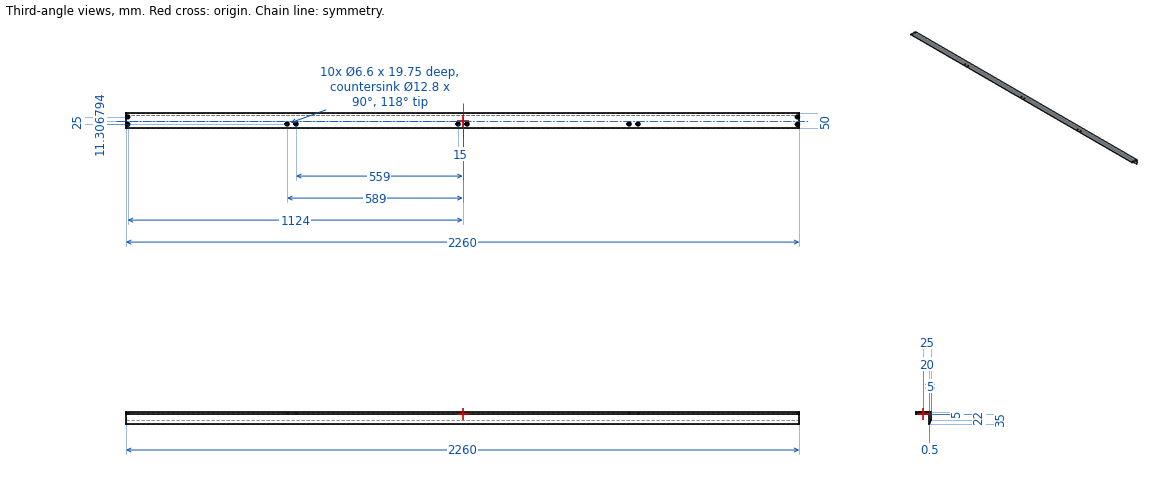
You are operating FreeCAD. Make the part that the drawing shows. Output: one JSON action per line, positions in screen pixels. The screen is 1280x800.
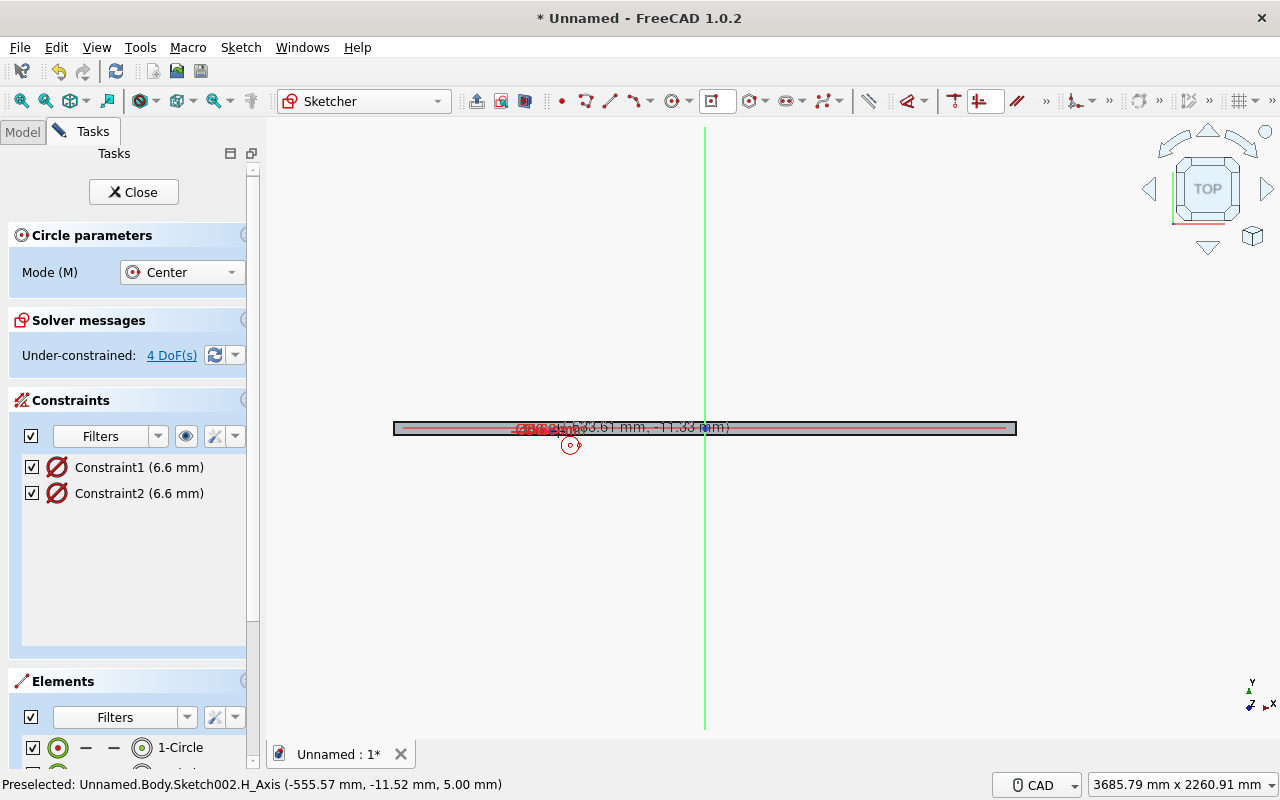
{"action": "scroll", "coordinate": [701, 432], "scroll_direction": "up", "scroll_amount": 17}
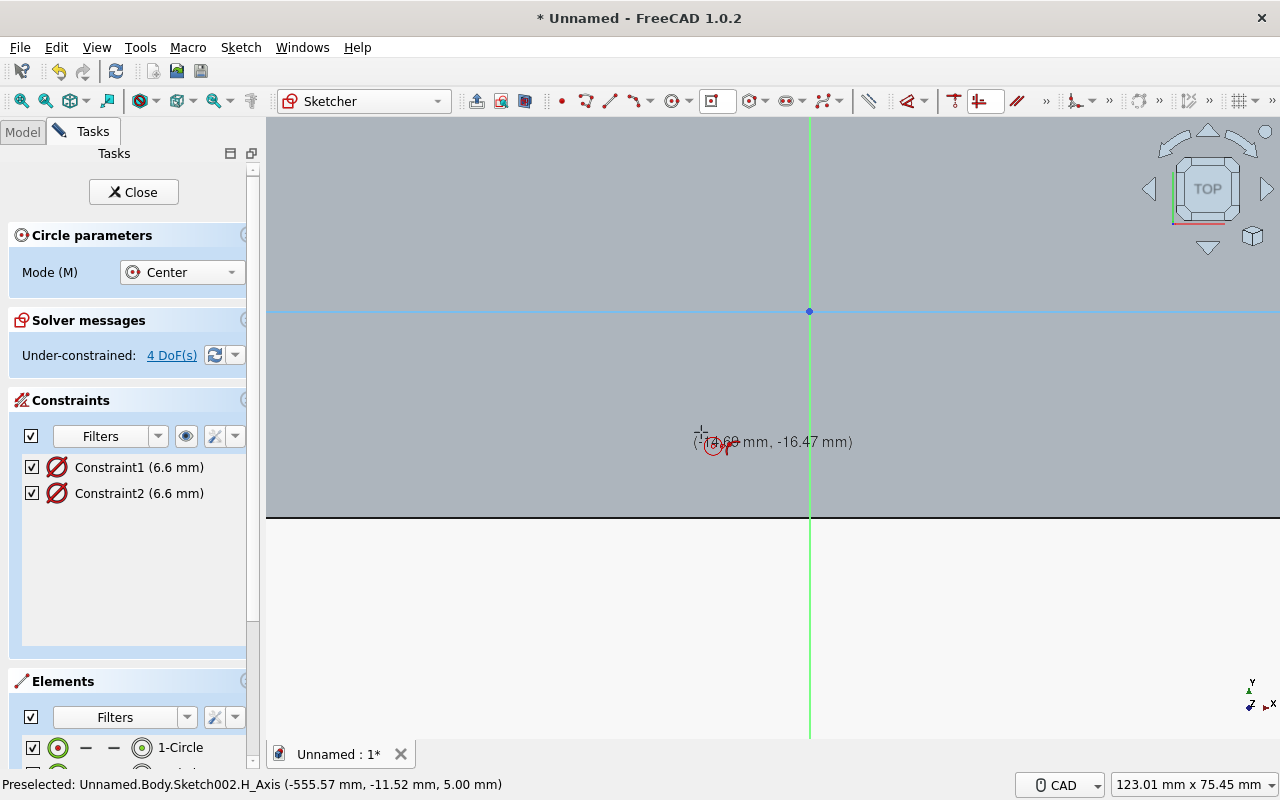
{"action": "scroll", "coordinate": [700, 433], "scroll_direction": "down", "scroll_amount": 16}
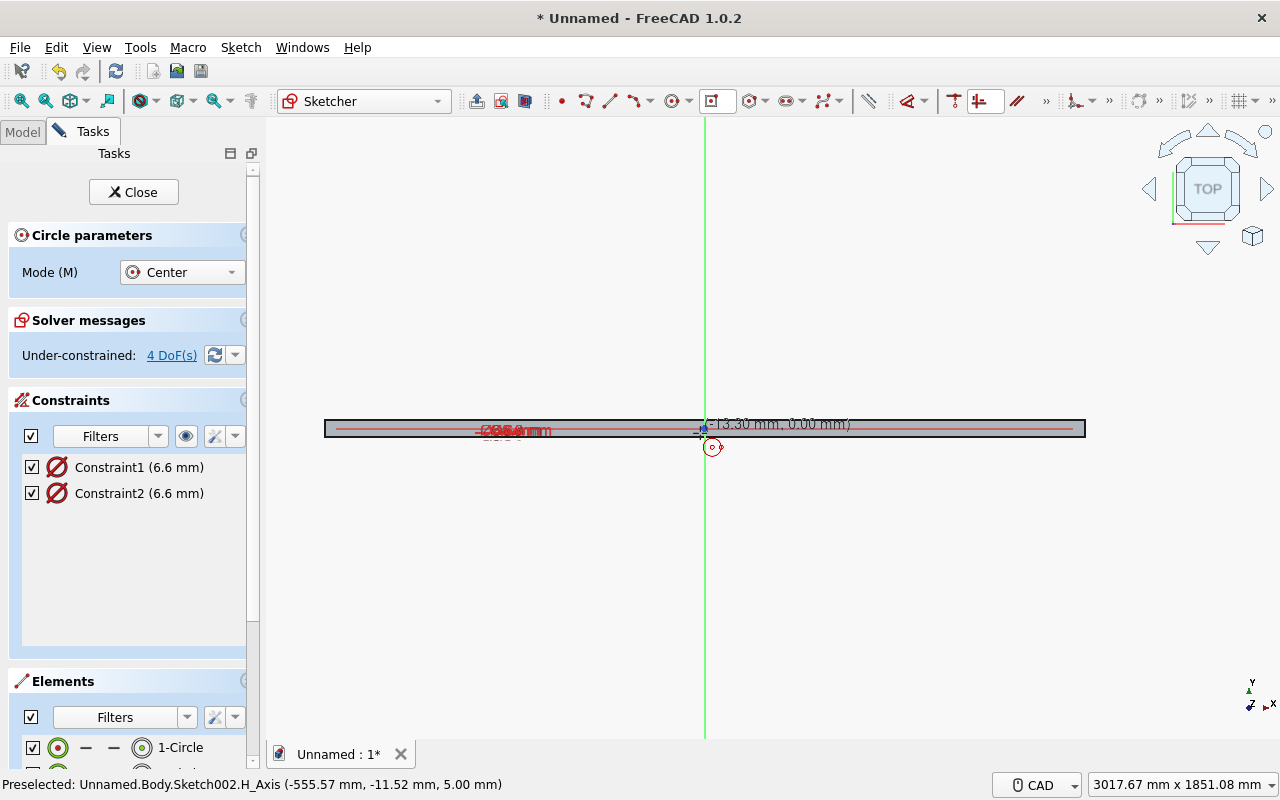
{"action": "scroll", "coordinate": [700, 432], "scroll_direction": "up", "scroll_amount": 8}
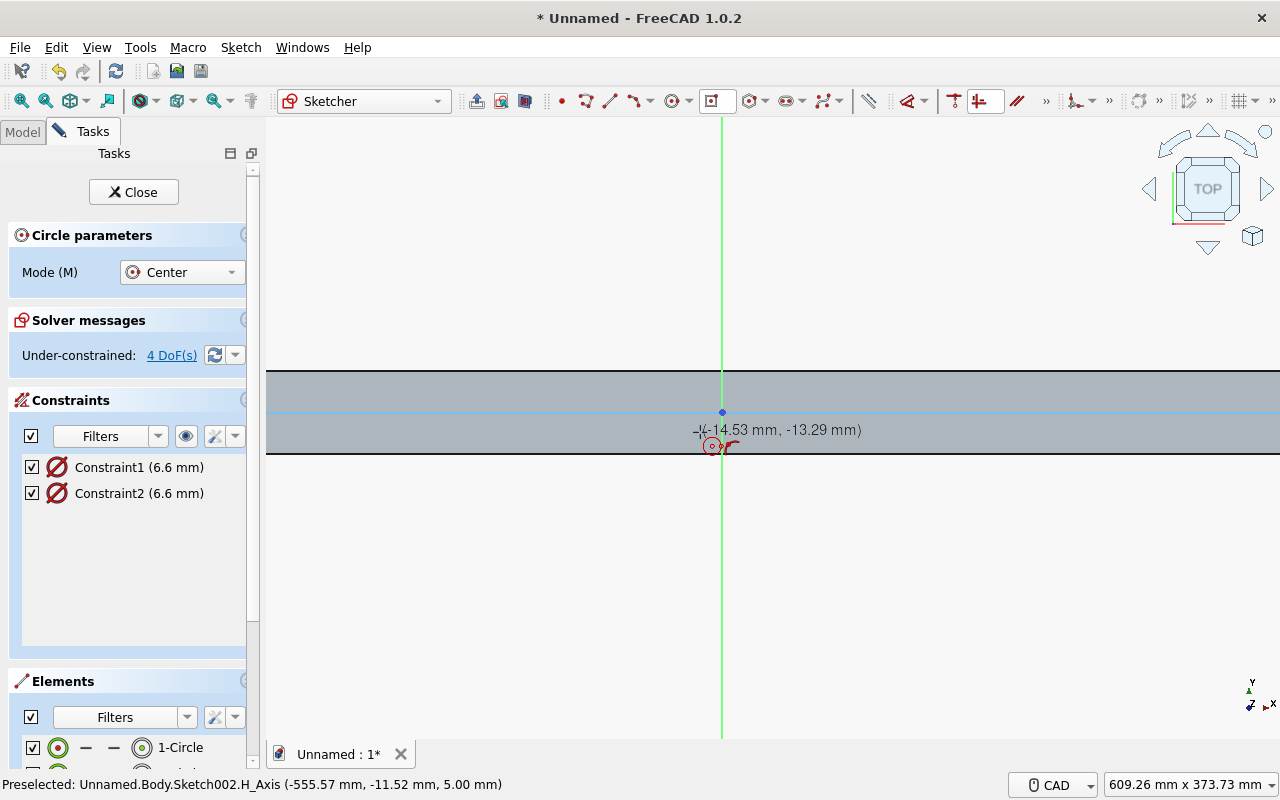
{"action": "left_click", "coordinate": [698, 432]}
{"action": "mouse_move", "coordinate": [701, 428]}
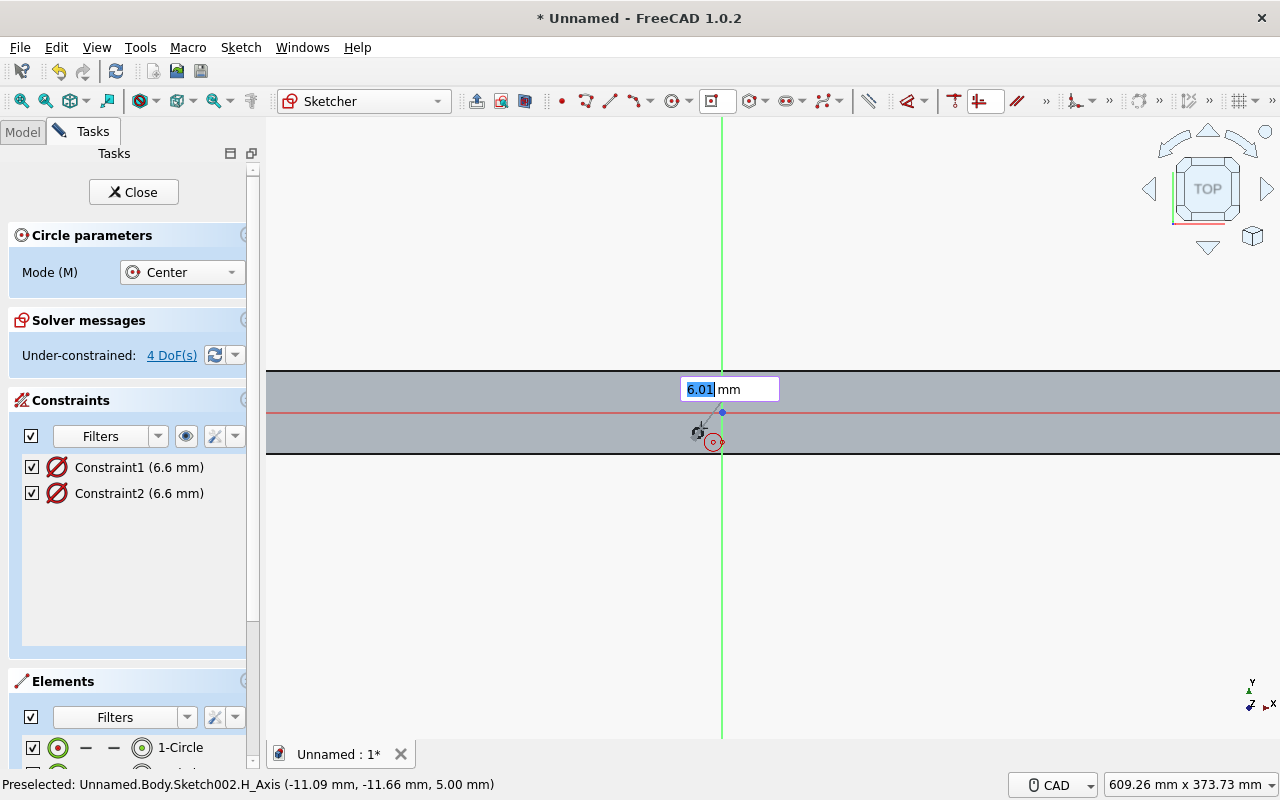
{"action": "type", "text": "6.6"}
{"action": "key", "text": "Return"}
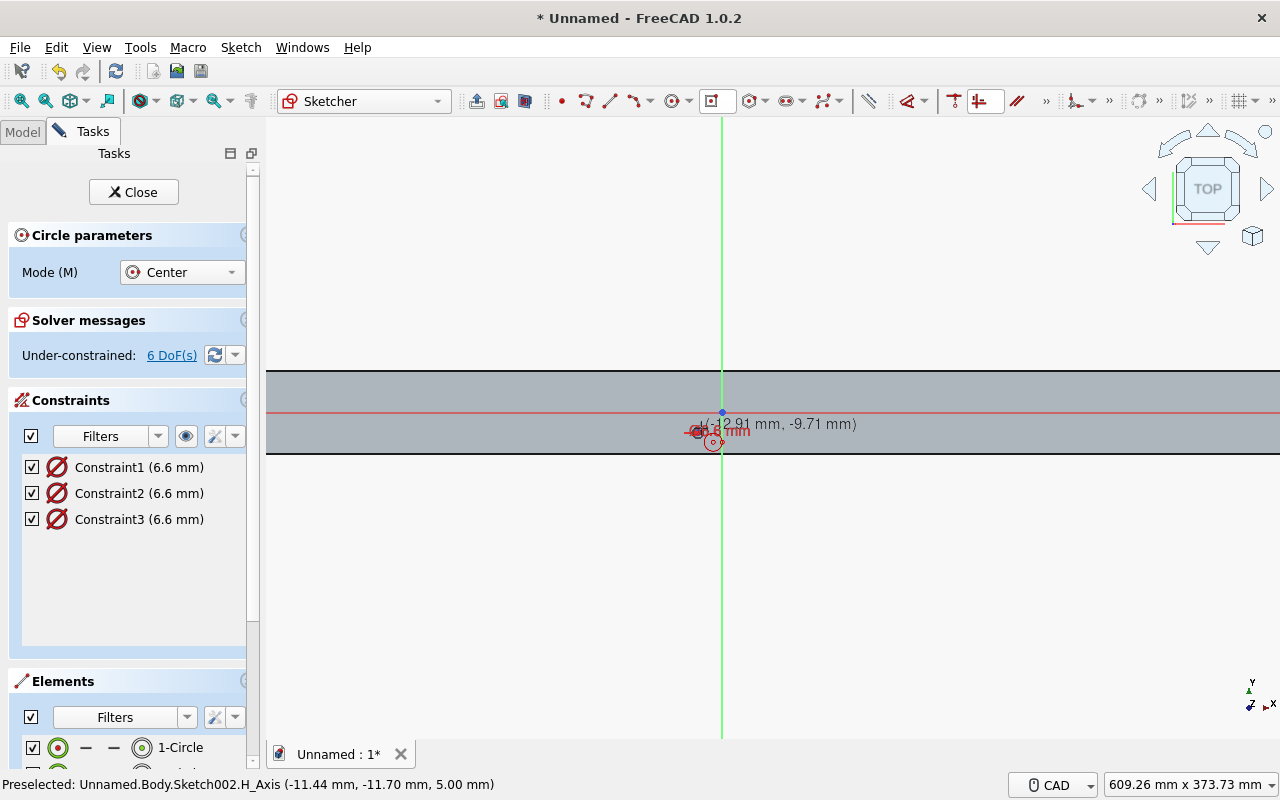
{"action": "scroll", "coordinate": [747, 432], "scroll_direction": "up", "scroll_amount": 8}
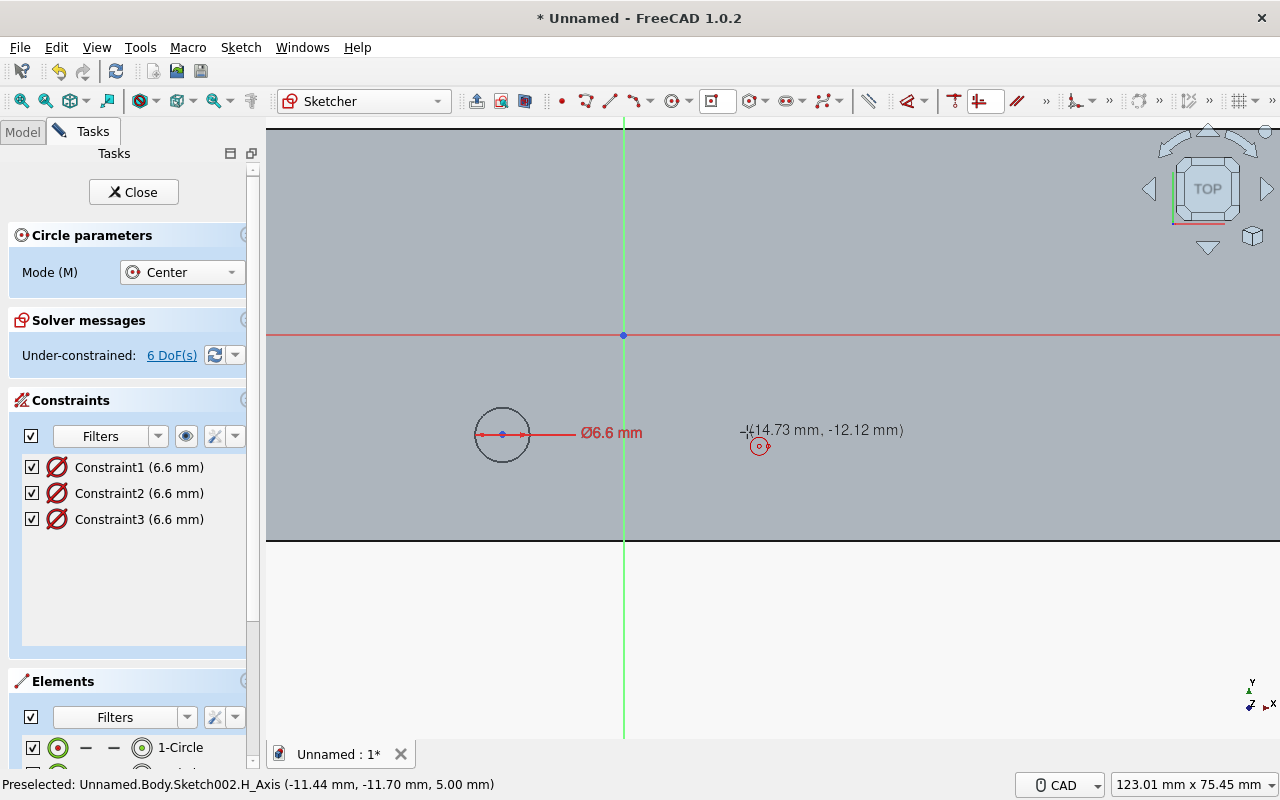
{"action": "scroll", "coordinate": [708, 432], "scroll_direction": "down", "scroll_amount": 16}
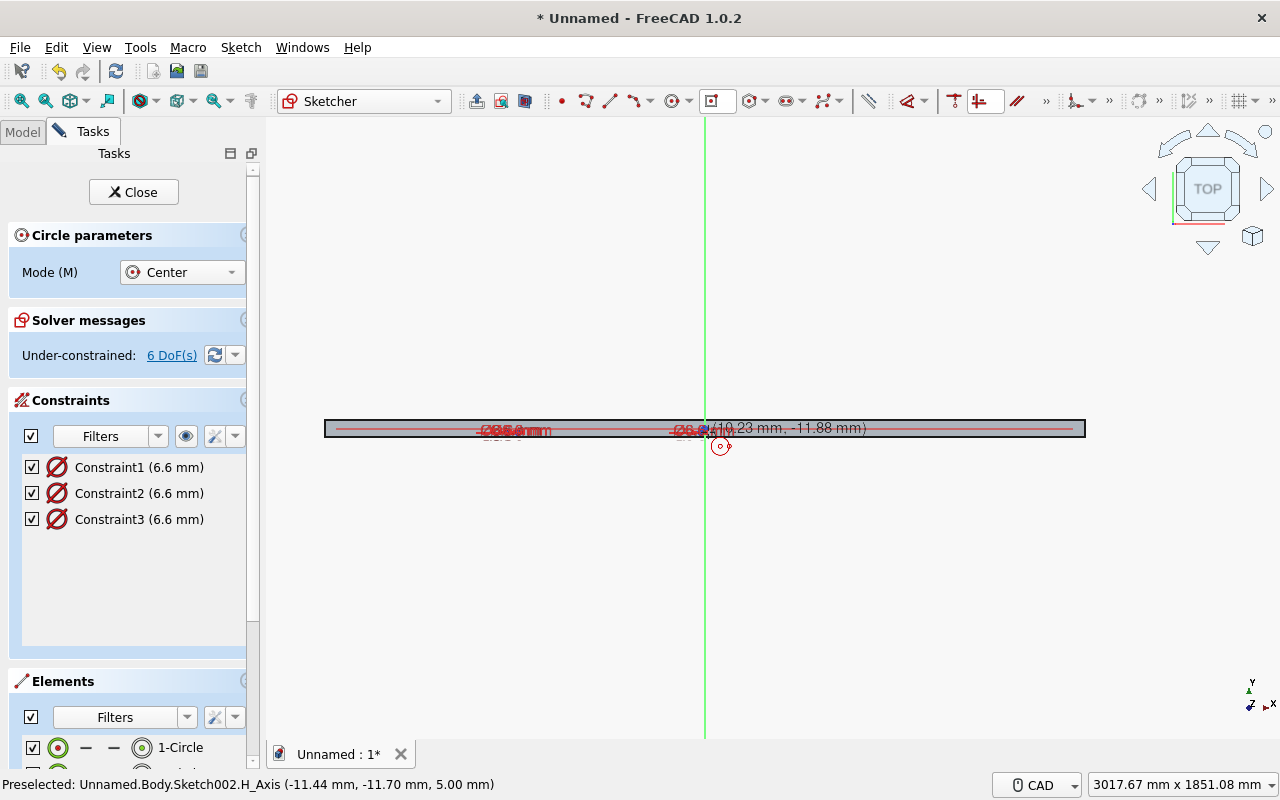
{"action": "scroll", "coordinate": [710, 432], "scroll_direction": "up", "scroll_amount": 8}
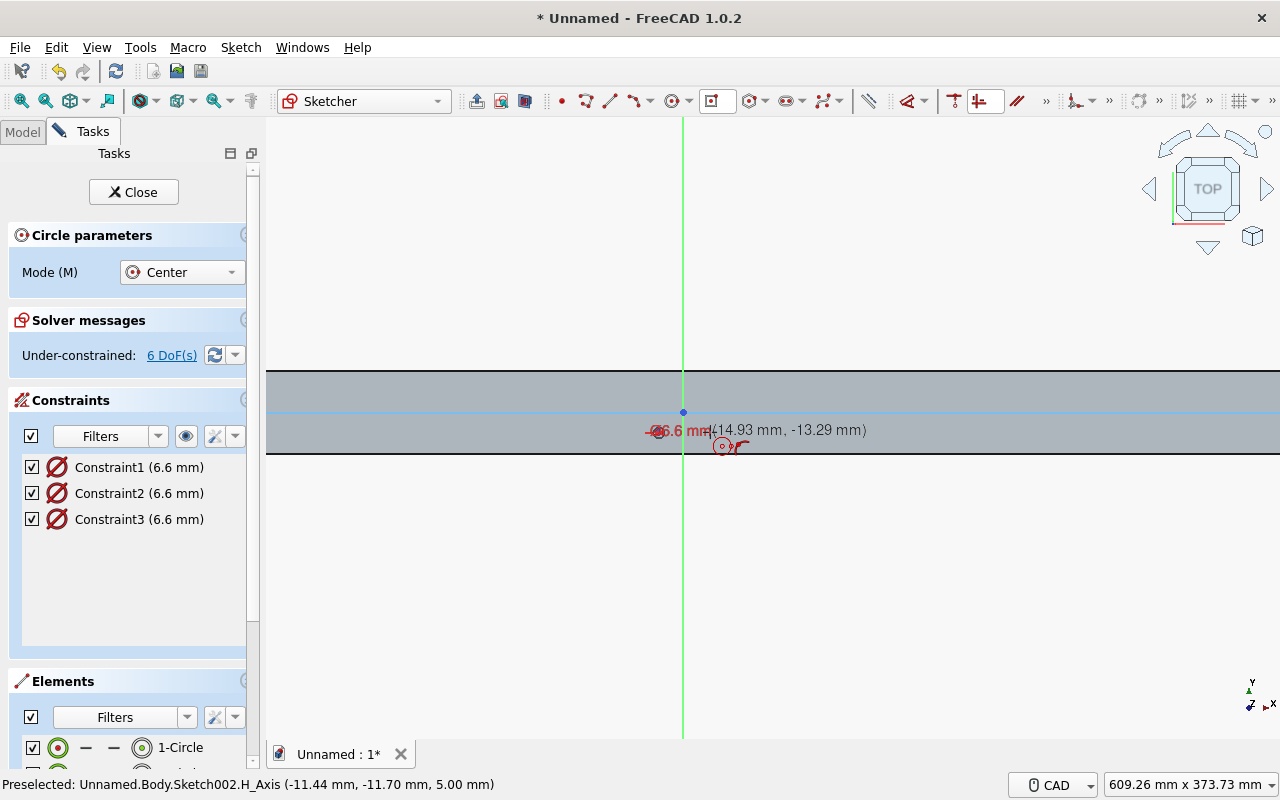
{"action": "left_click", "coordinate": [708, 432]}
{"action": "mouse_move", "coordinate": [712, 428]}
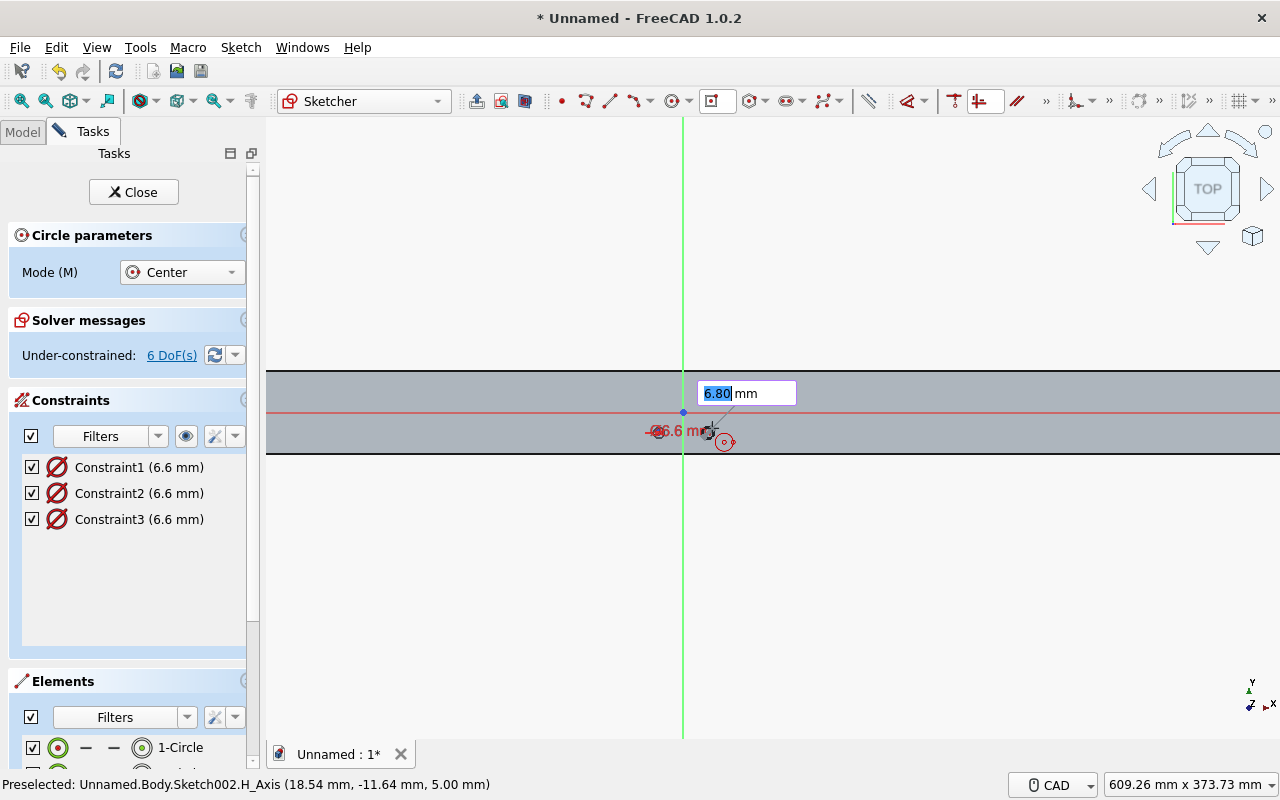
{"action": "type", "text": "6.6"}
{"action": "key", "text": "Return"}